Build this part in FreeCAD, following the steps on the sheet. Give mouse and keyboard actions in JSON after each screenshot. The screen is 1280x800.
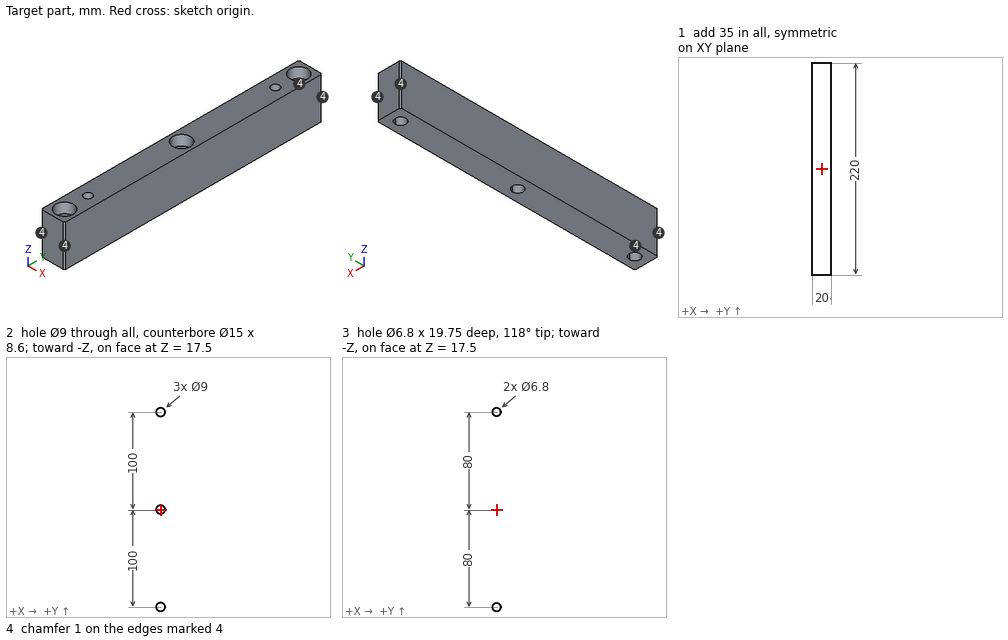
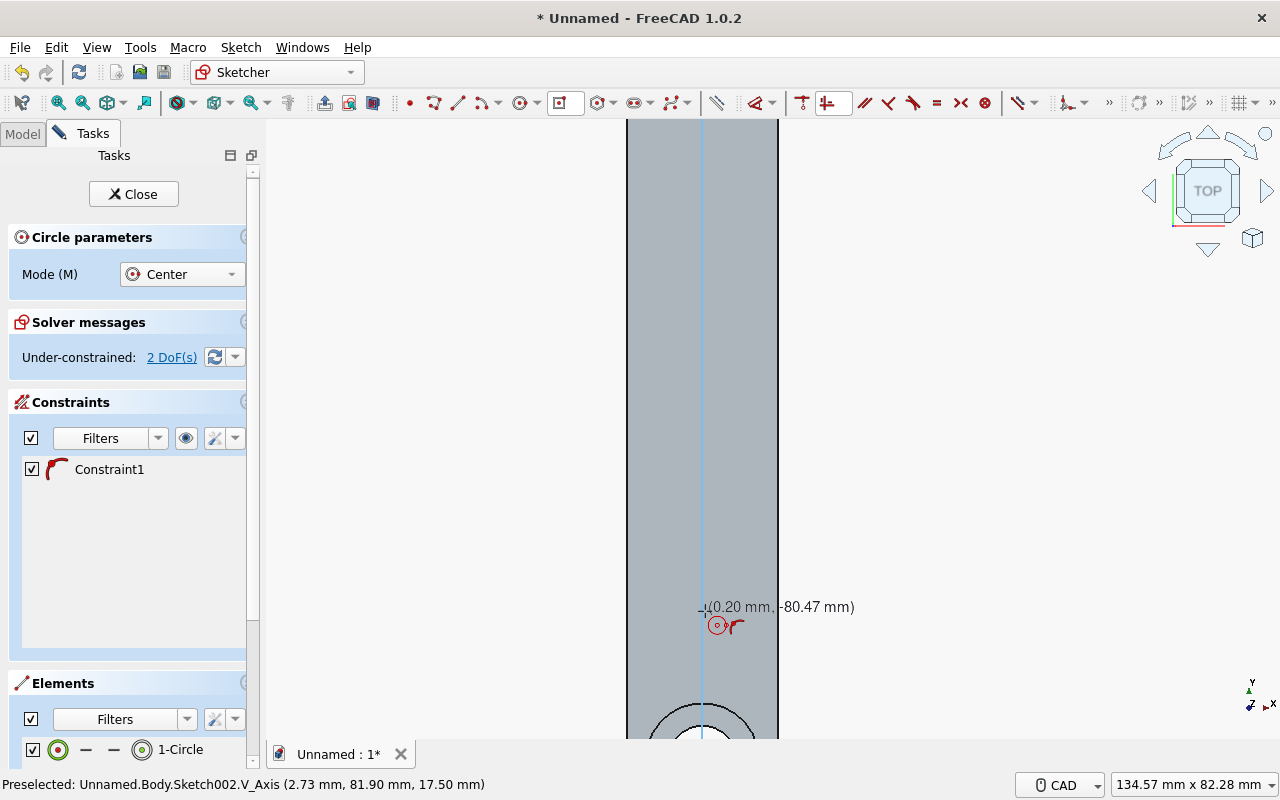
{"action": "left_click", "coordinate": [702, 609]}
{"action": "left_click", "coordinate": [721, 591]}
{"action": "key", "text": "Escape"}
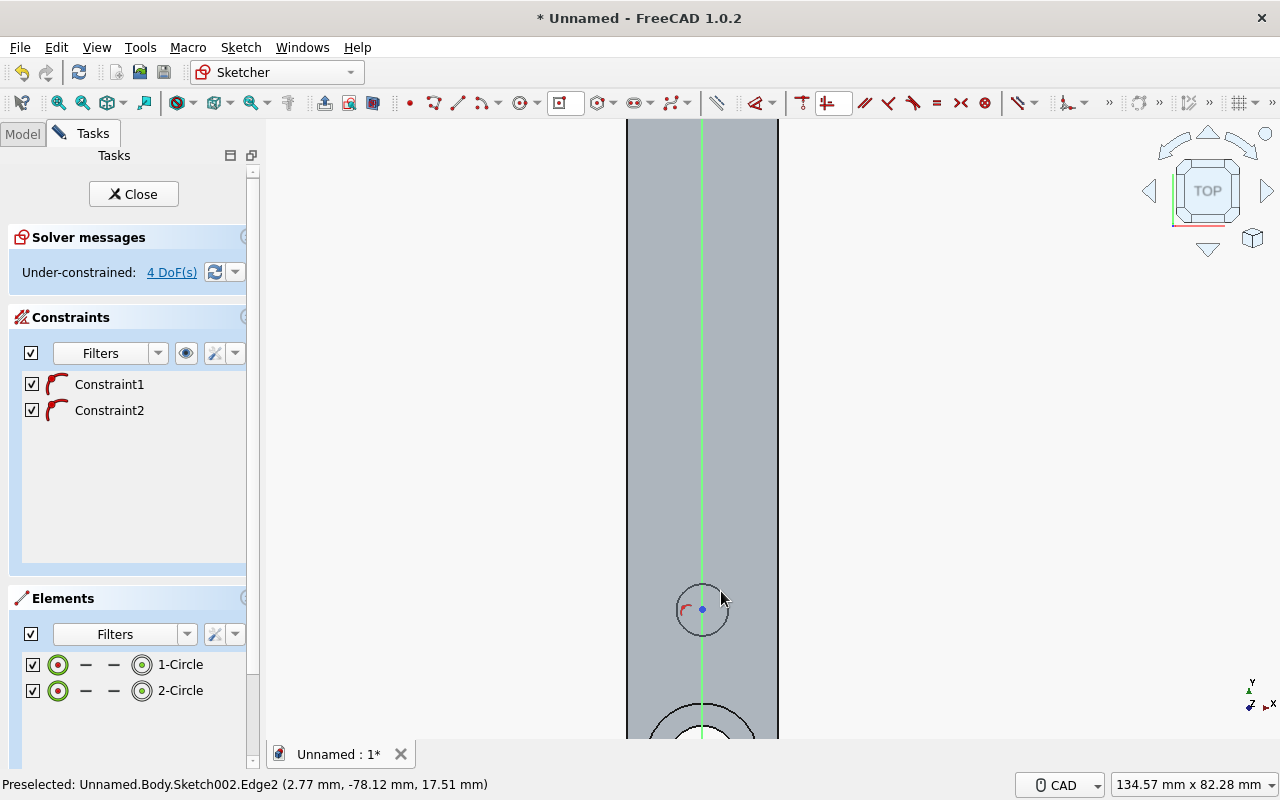
{"action": "scroll", "coordinate": [705, 611], "scroll_direction": "down", "scroll_amount": 6}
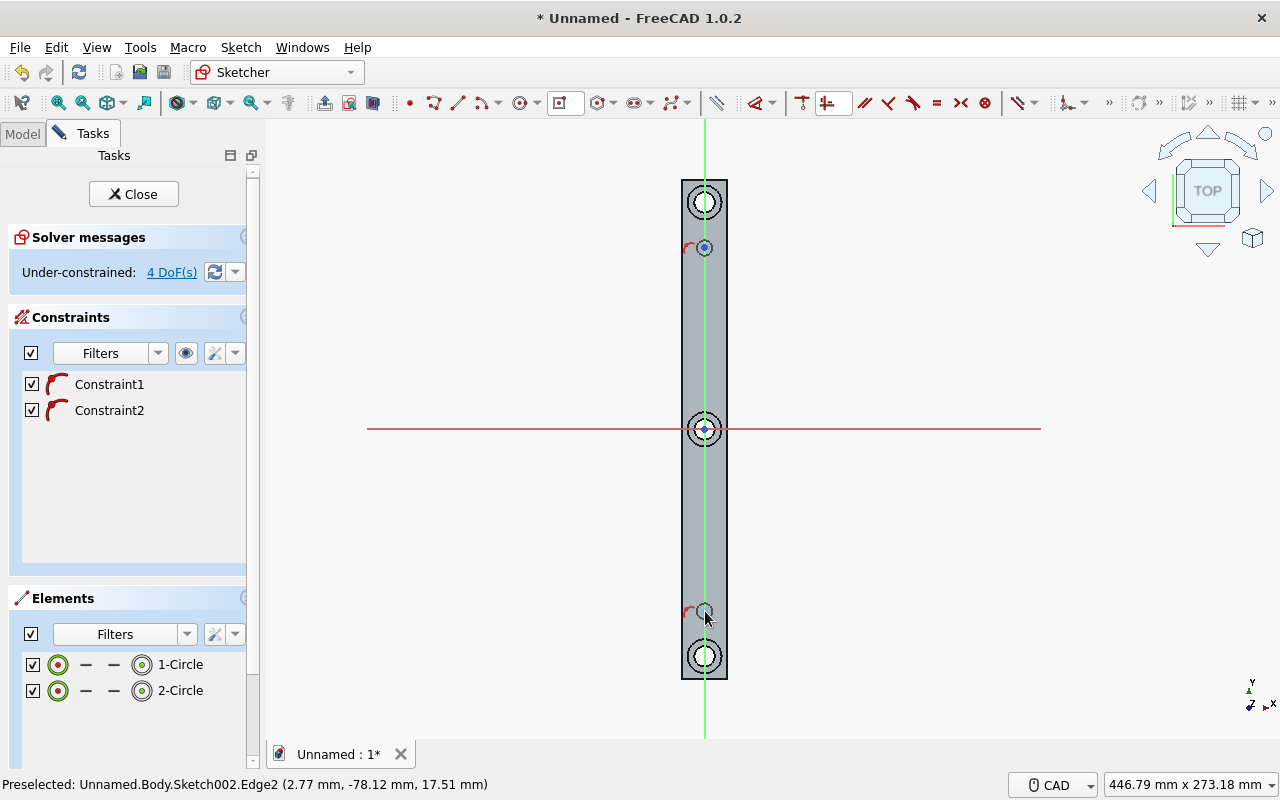
{"action": "scroll", "coordinate": [710, 243], "scroll_direction": "up", "scroll_amount": 5}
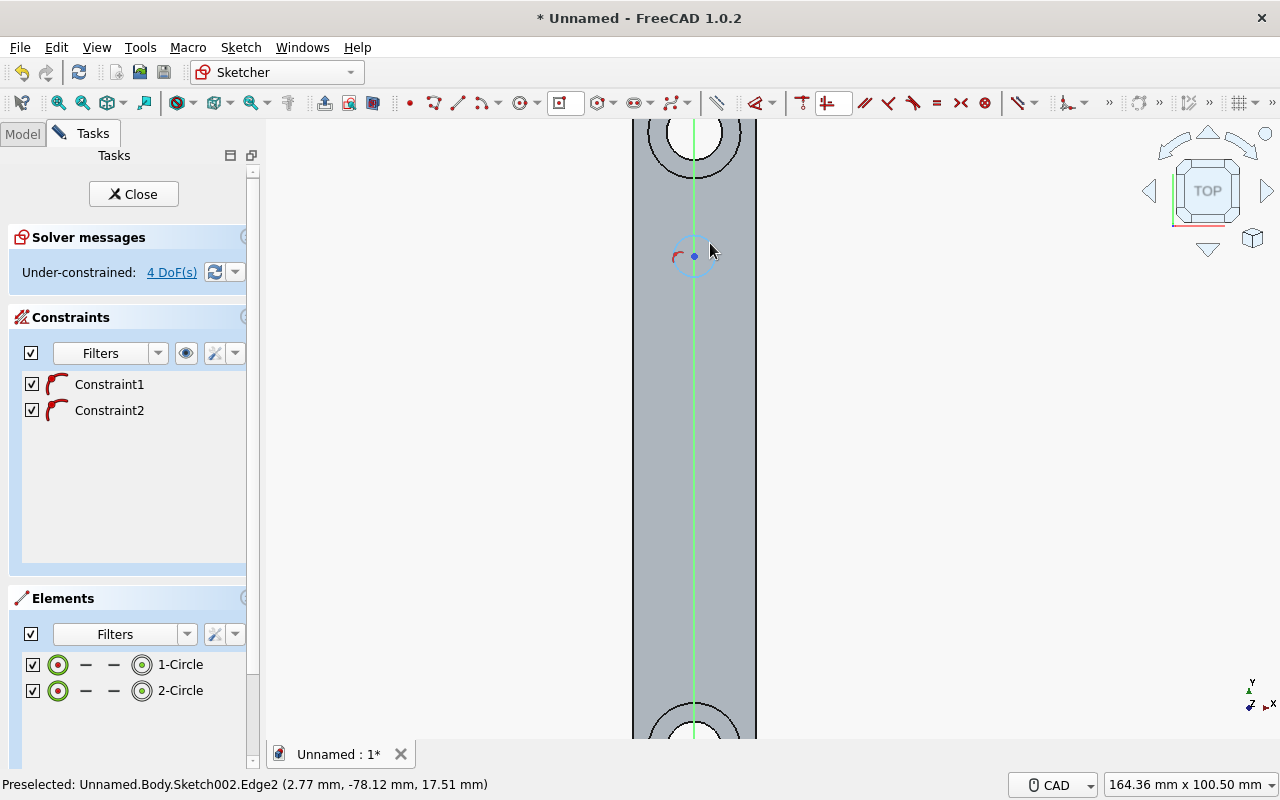
{"action": "left_click", "coordinate": [709, 242]}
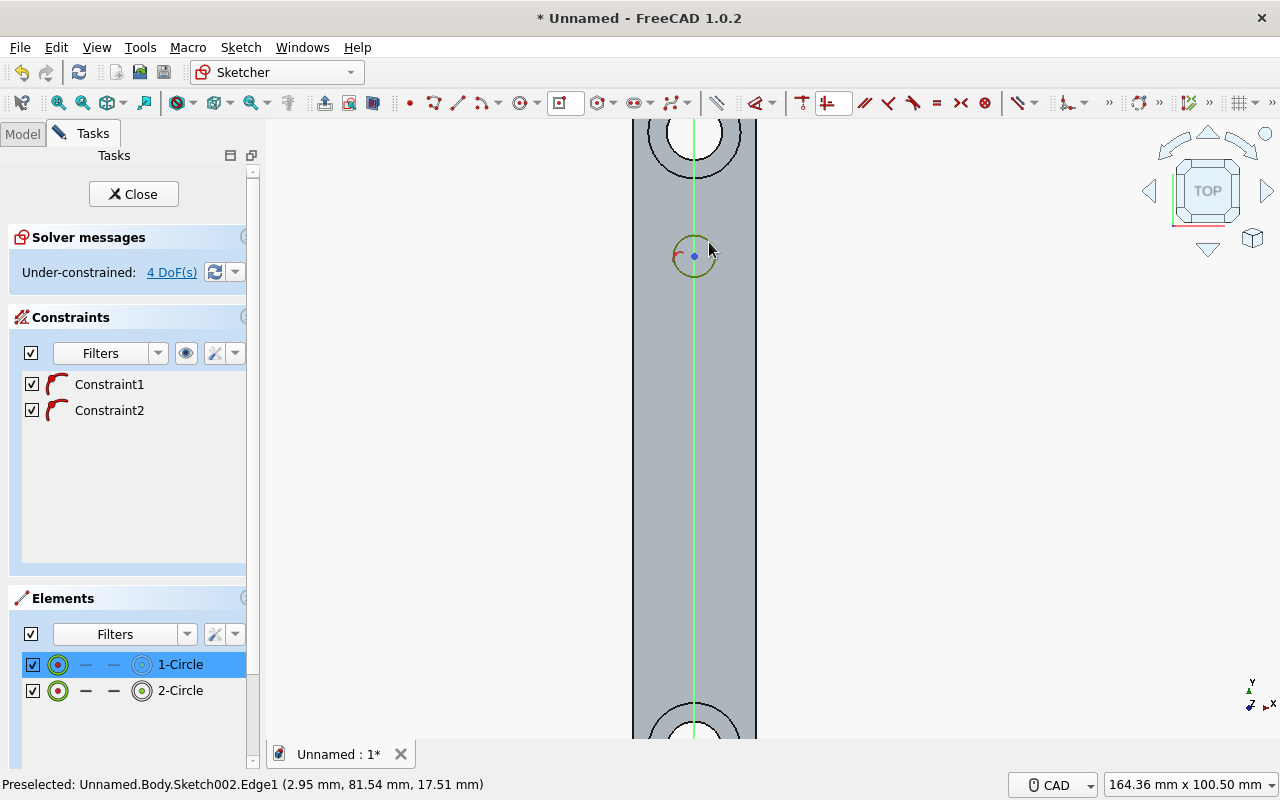
{"action": "scroll", "coordinate": [710, 243], "scroll_direction": "down", "scroll_amount": 5}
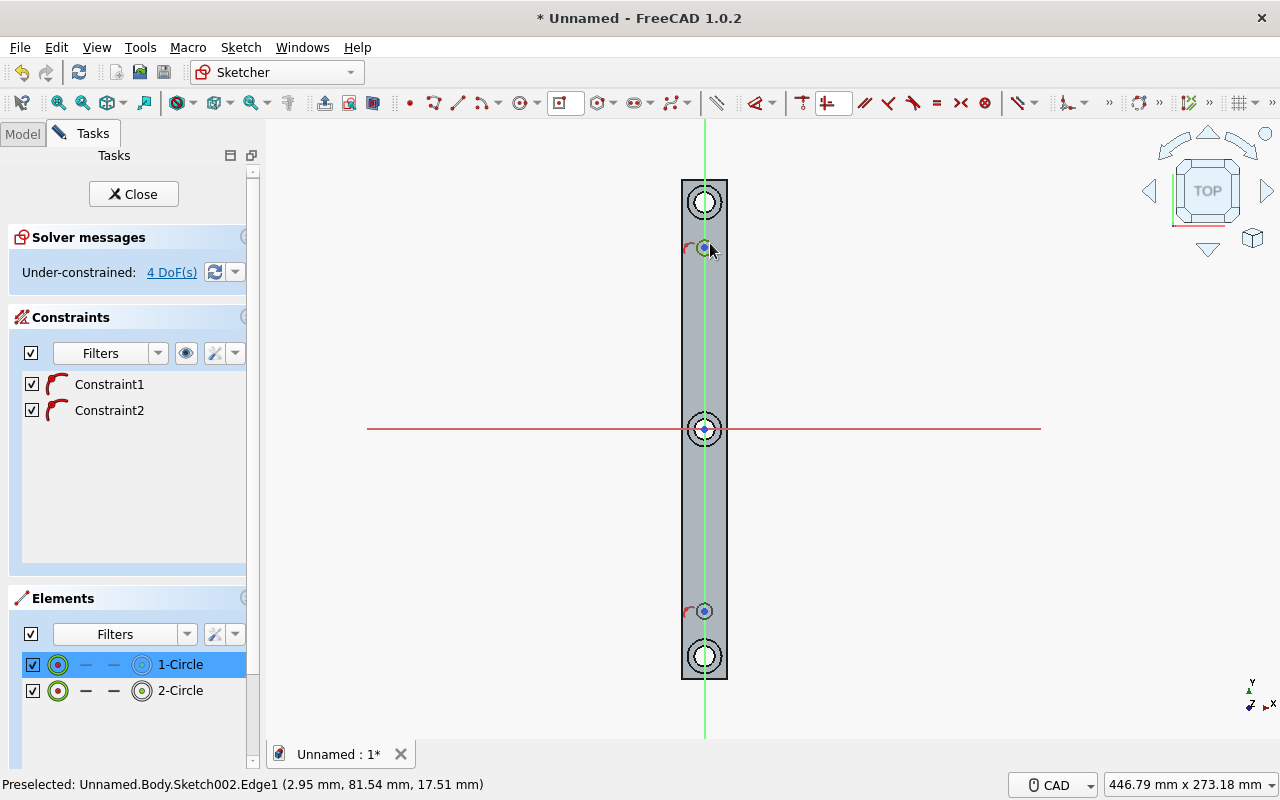
{"action": "scroll", "coordinate": [710, 606], "scroll_direction": "up", "scroll_amount": 5}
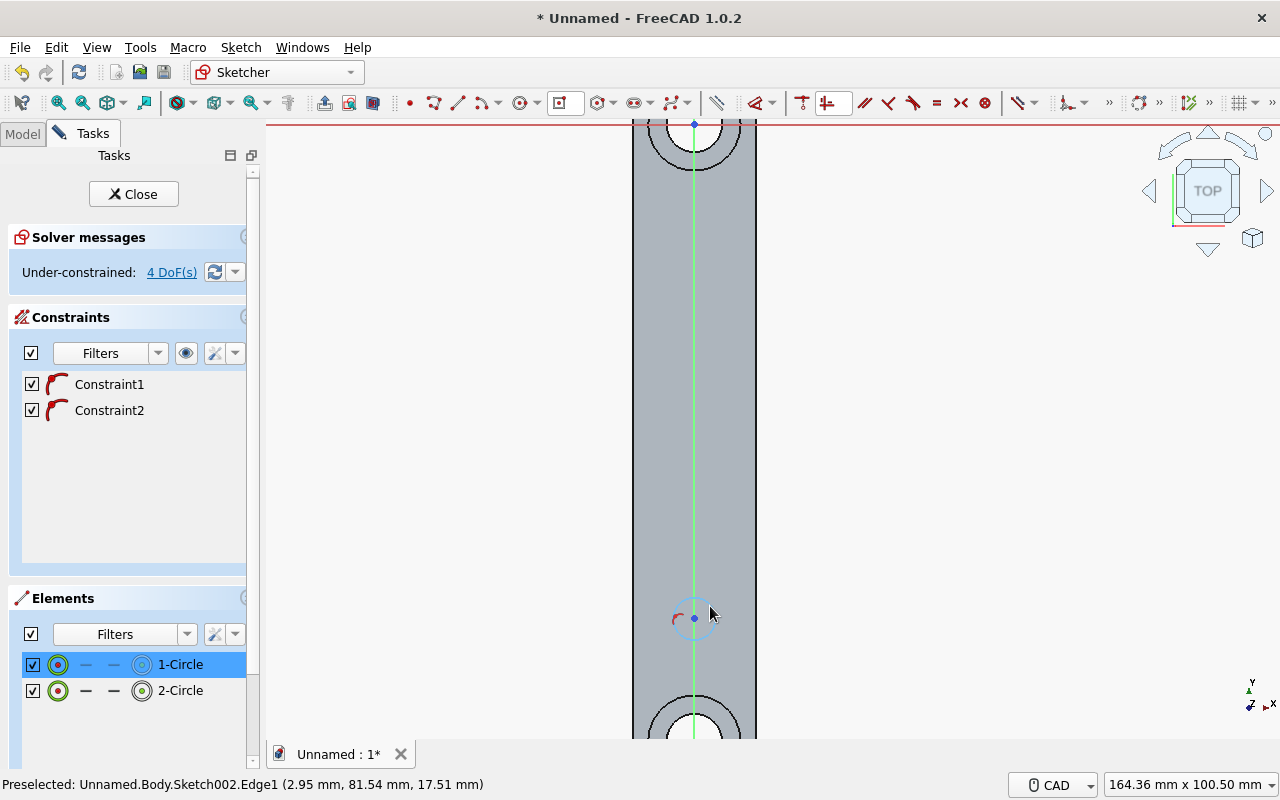
{"action": "left_click", "coordinate": [709, 604]}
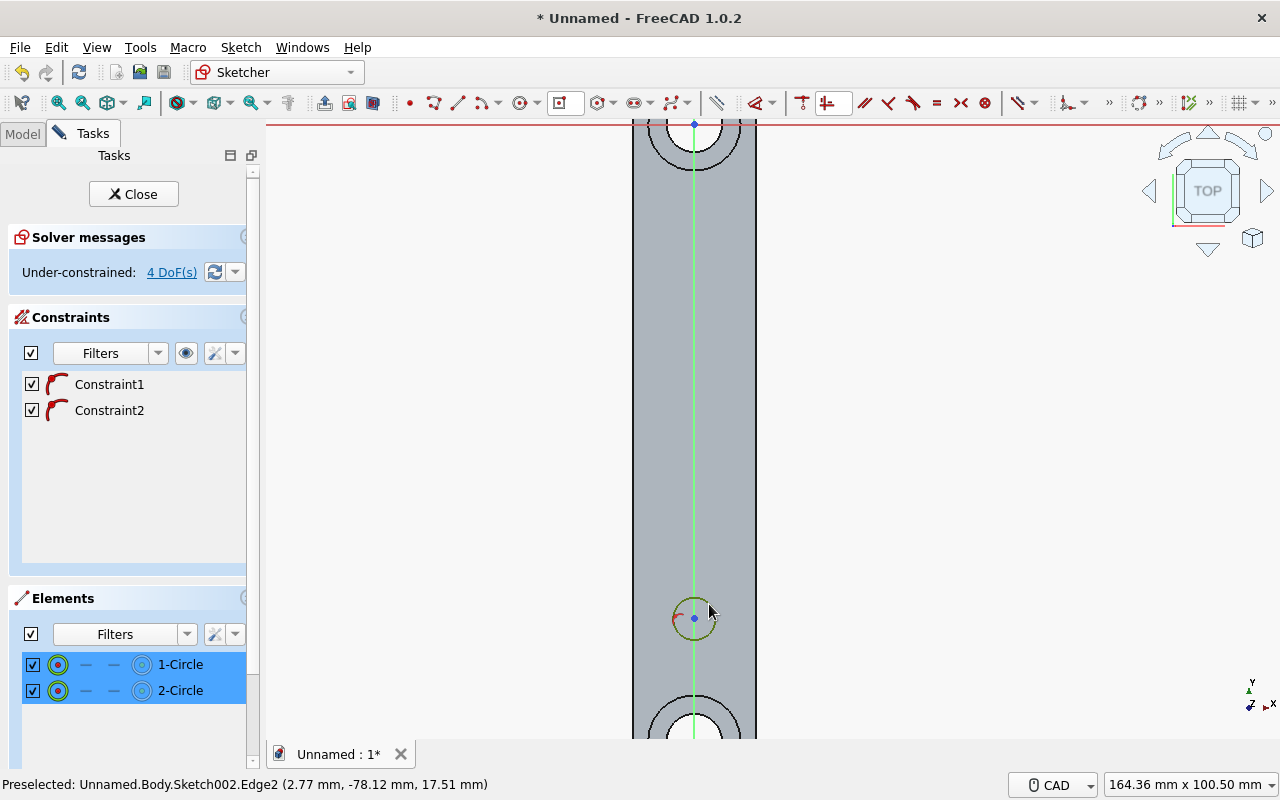
{"action": "left_click", "coordinate": [938, 104]}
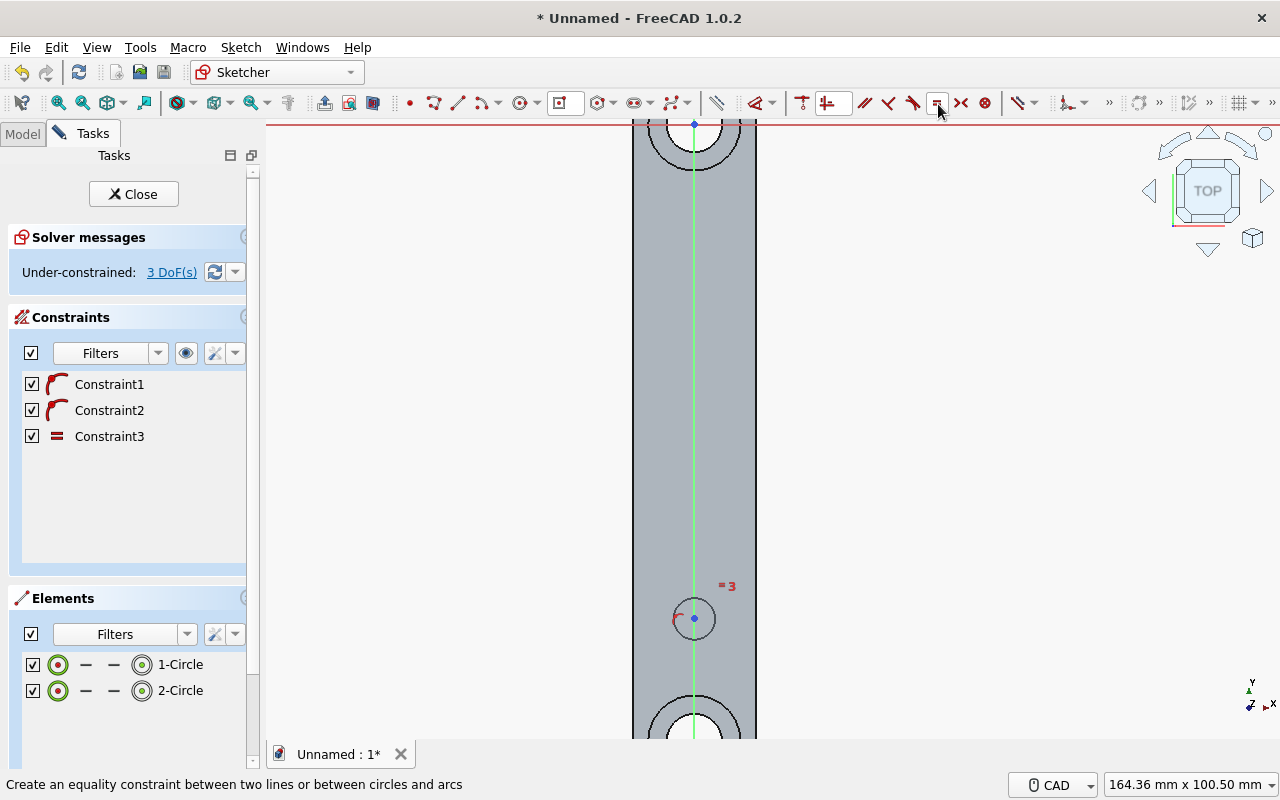
{"action": "left_click", "coordinate": [756, 104]}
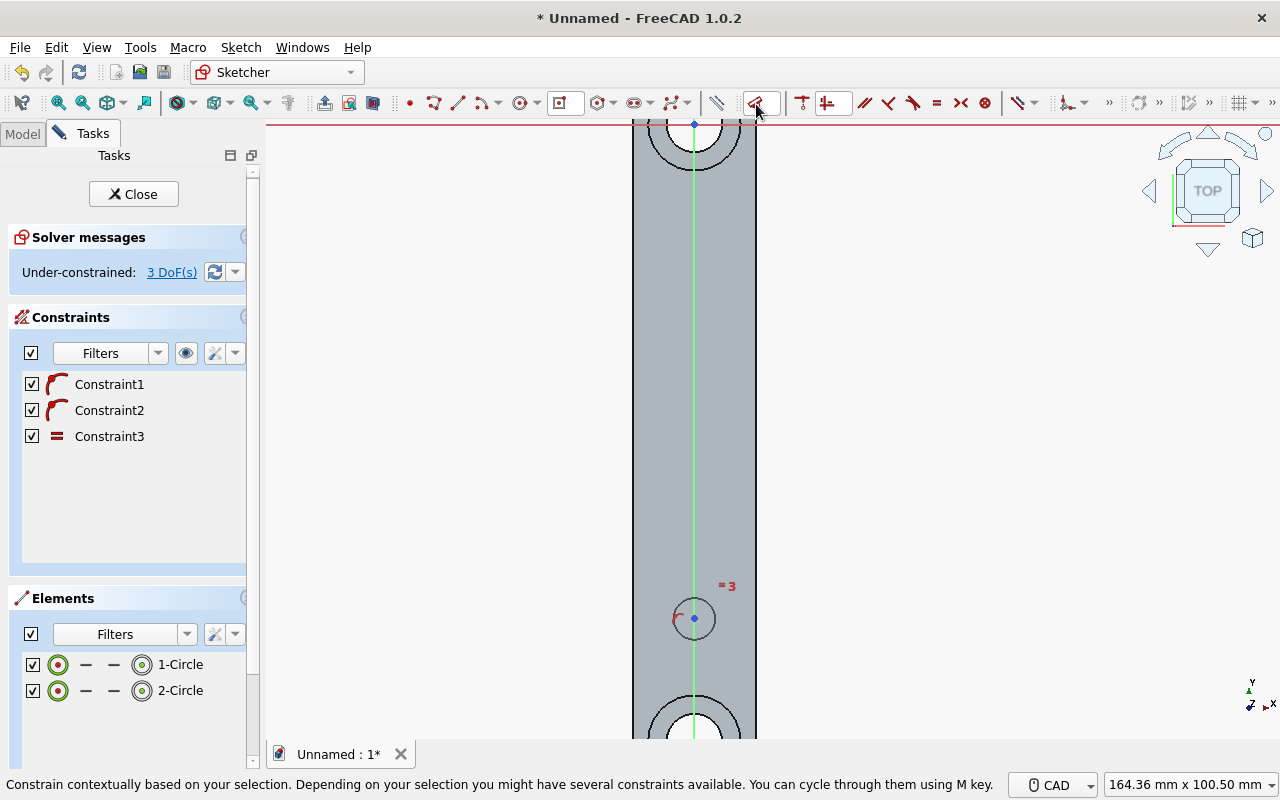
{"action": "scroll", "coordinate": [710, 606], "scroll_direction": "down", "scroll_amount": 5}